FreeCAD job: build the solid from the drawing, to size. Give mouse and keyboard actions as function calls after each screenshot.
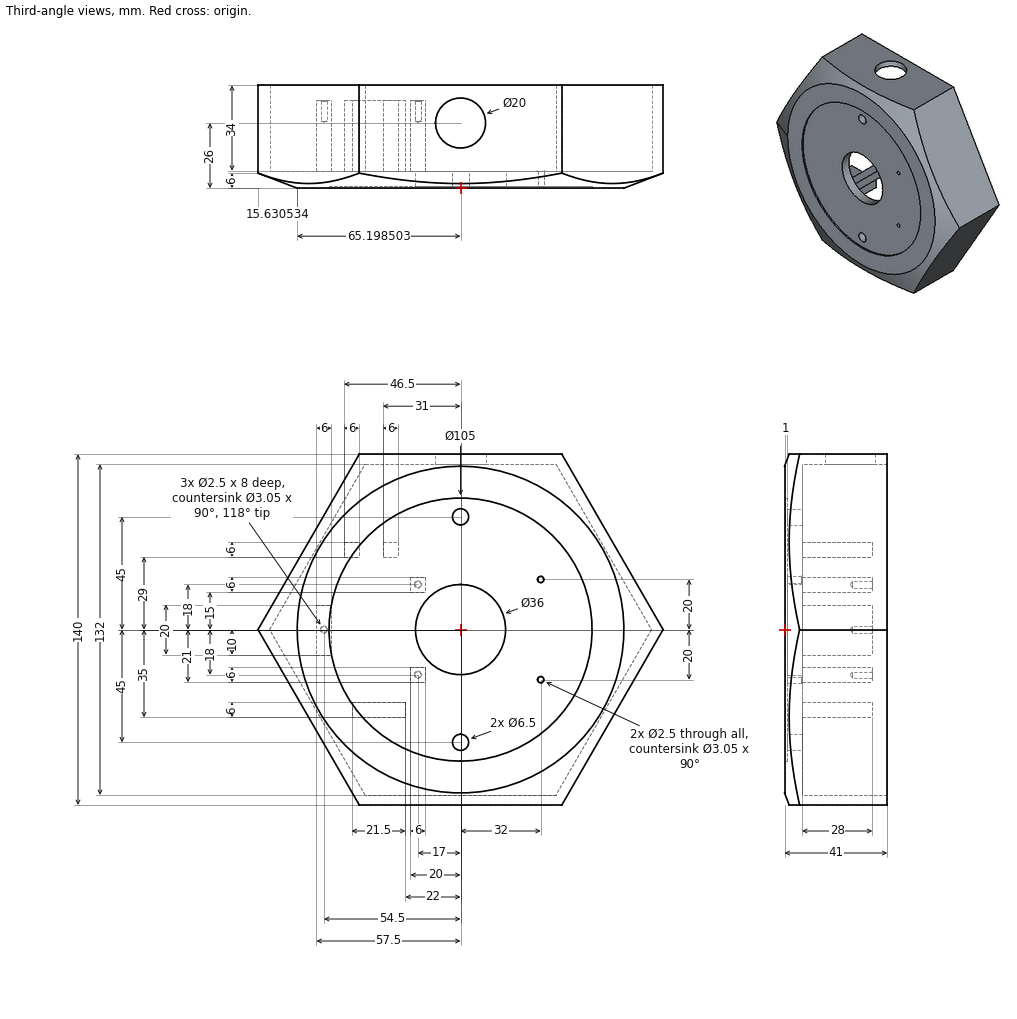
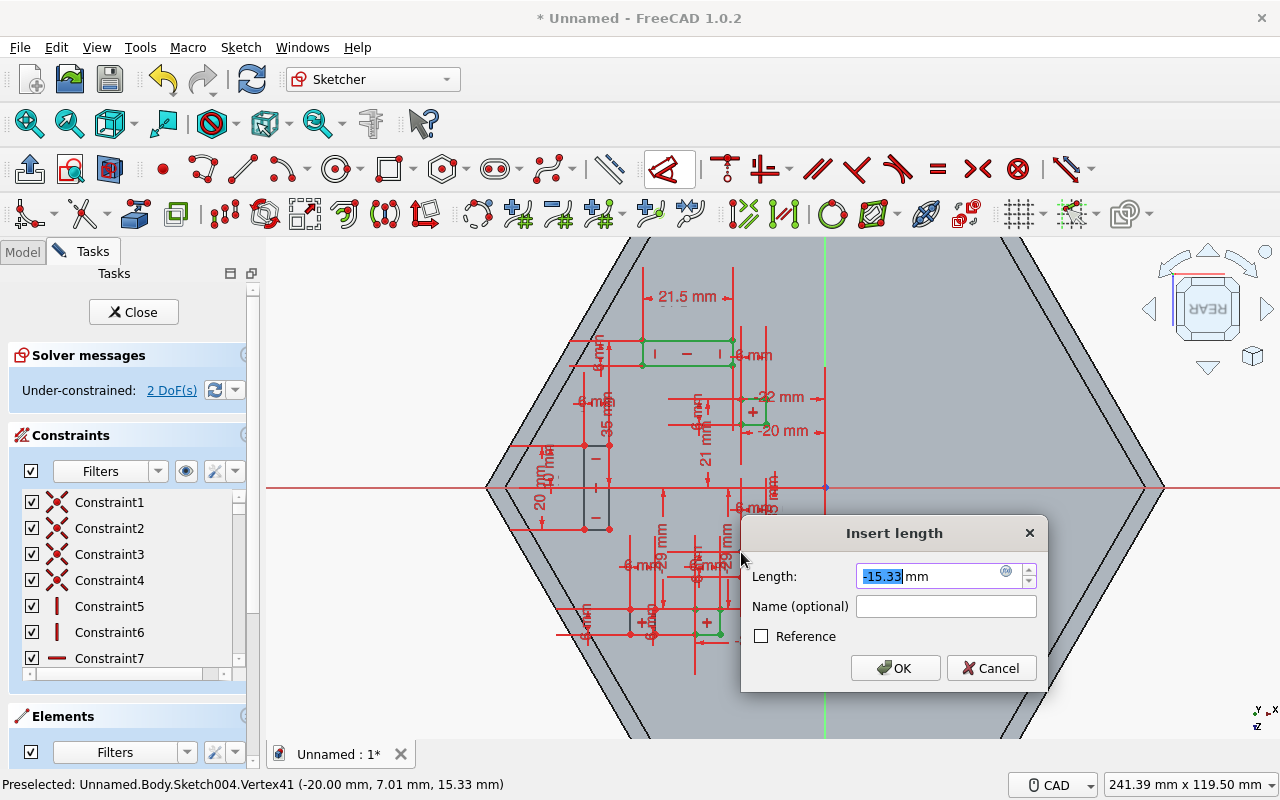
text(-15)
key(Return)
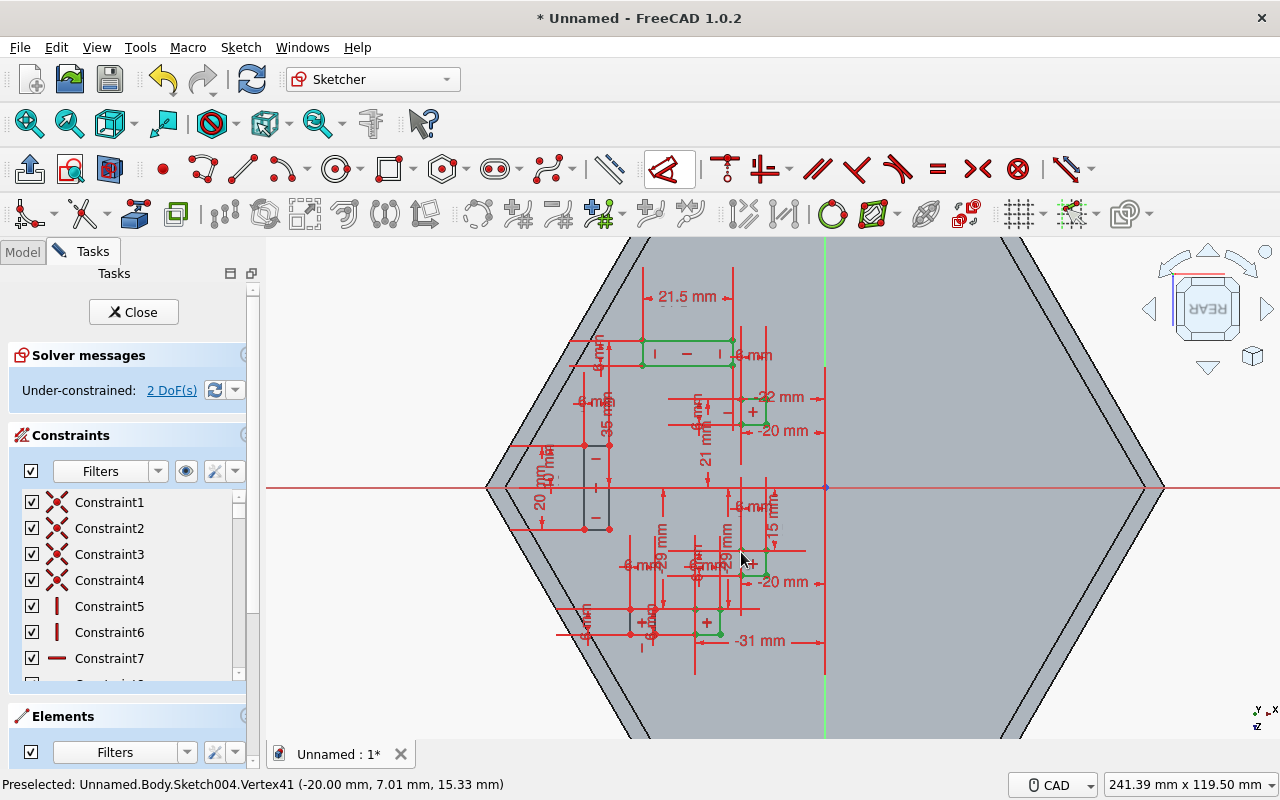
click(584, 446)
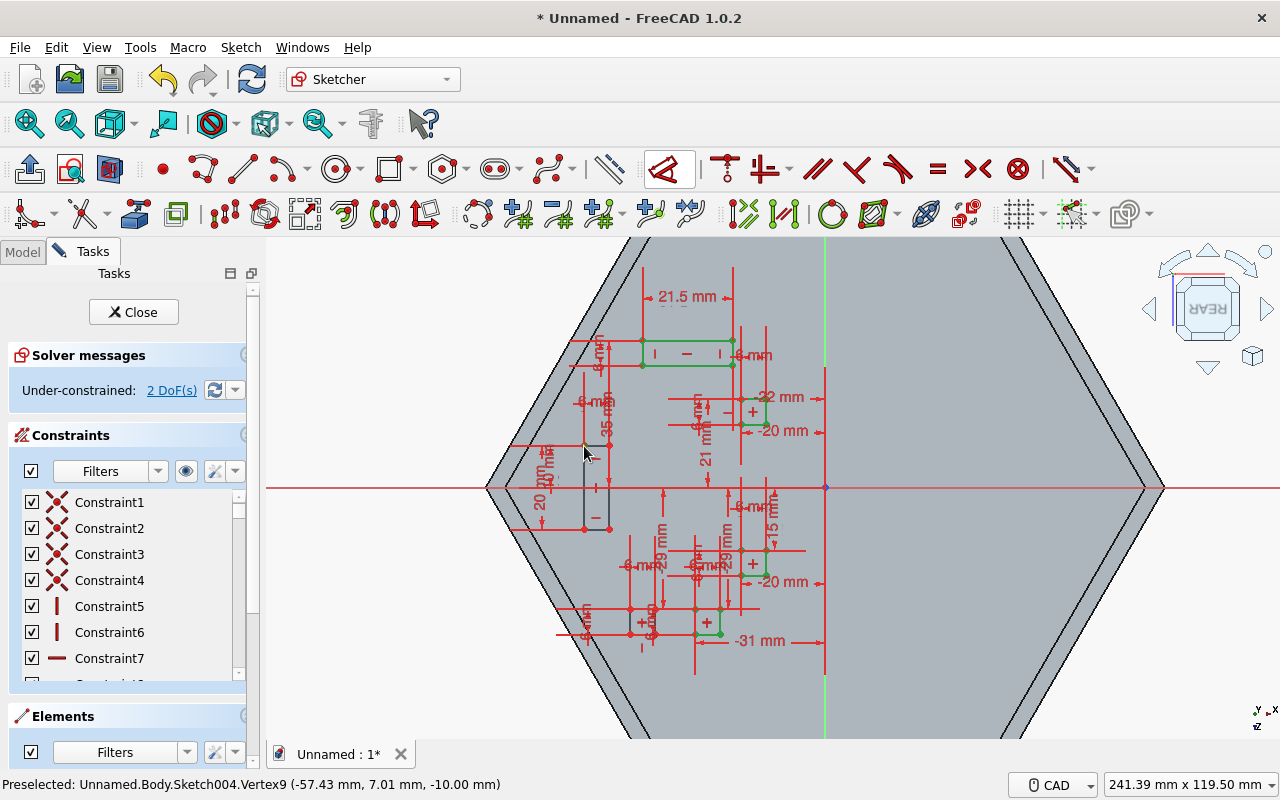
key(l)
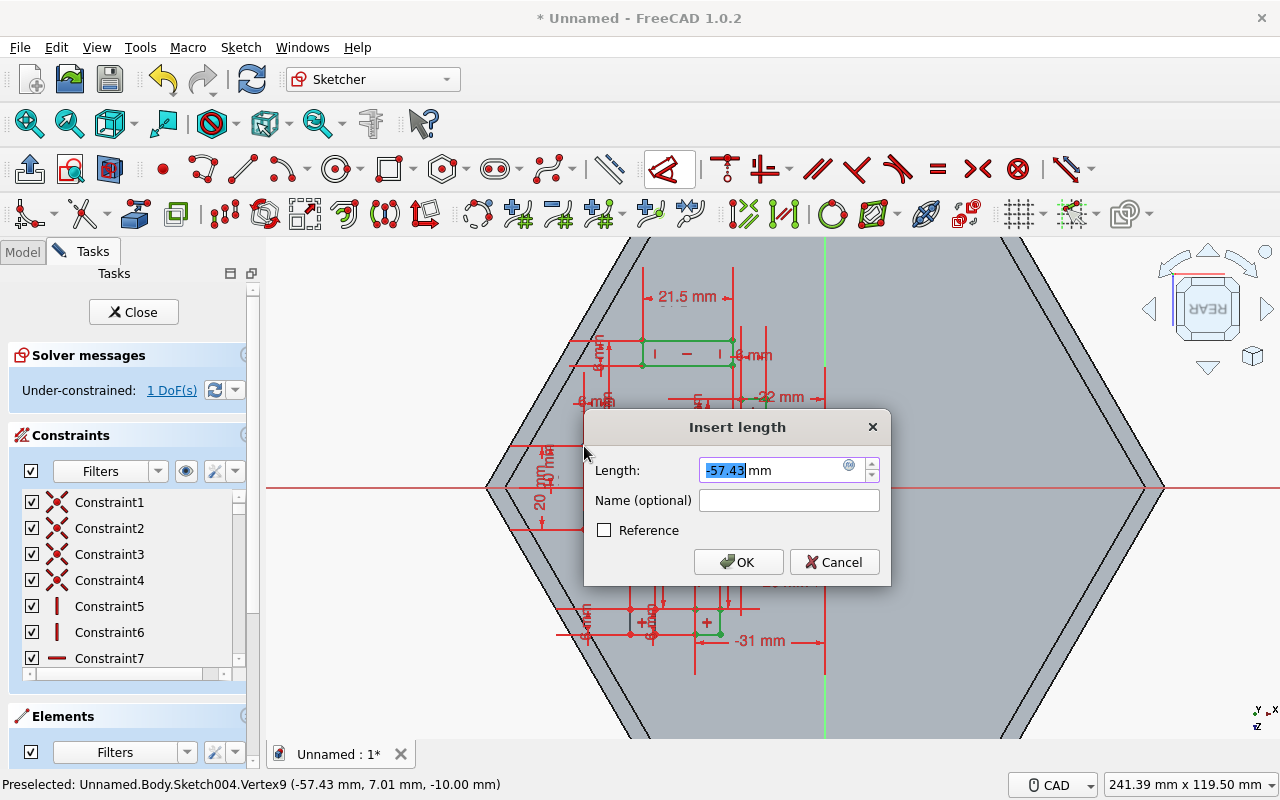
text(-57.5)
key(Return)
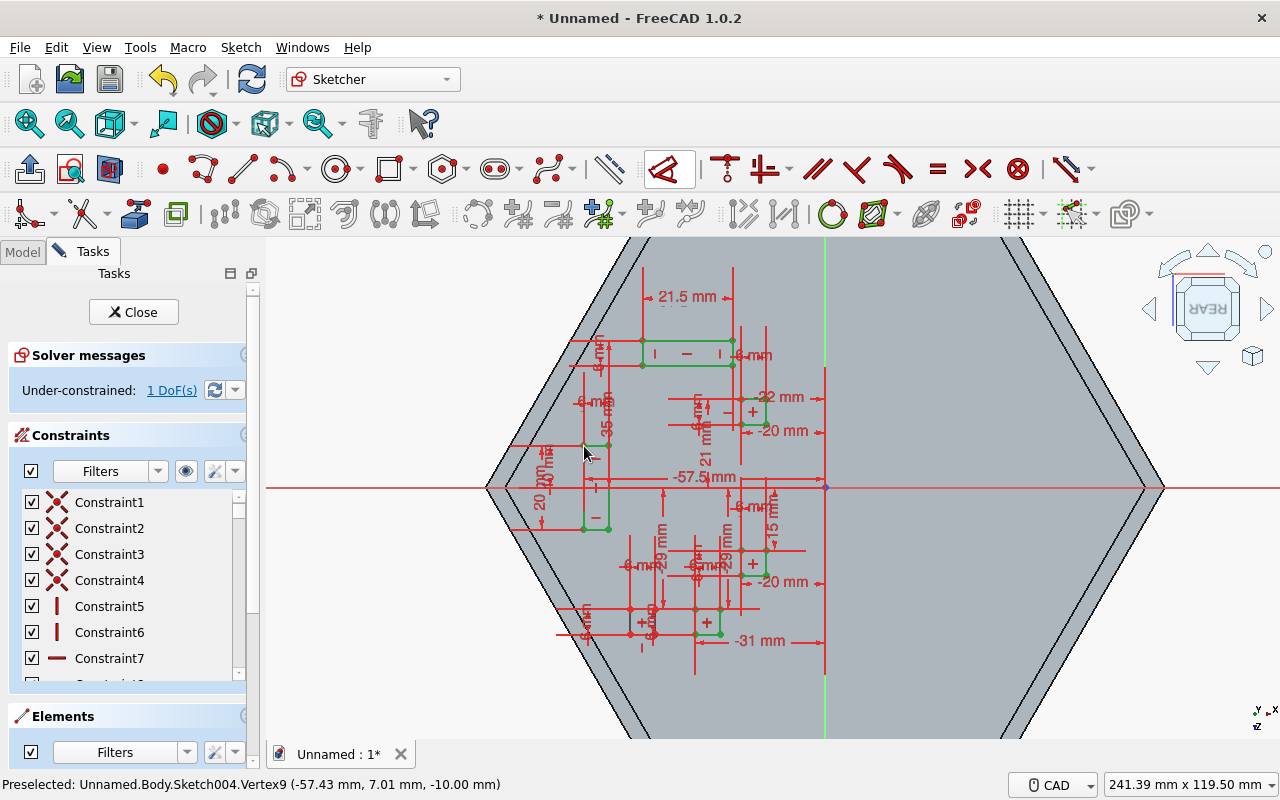
click(630, 609)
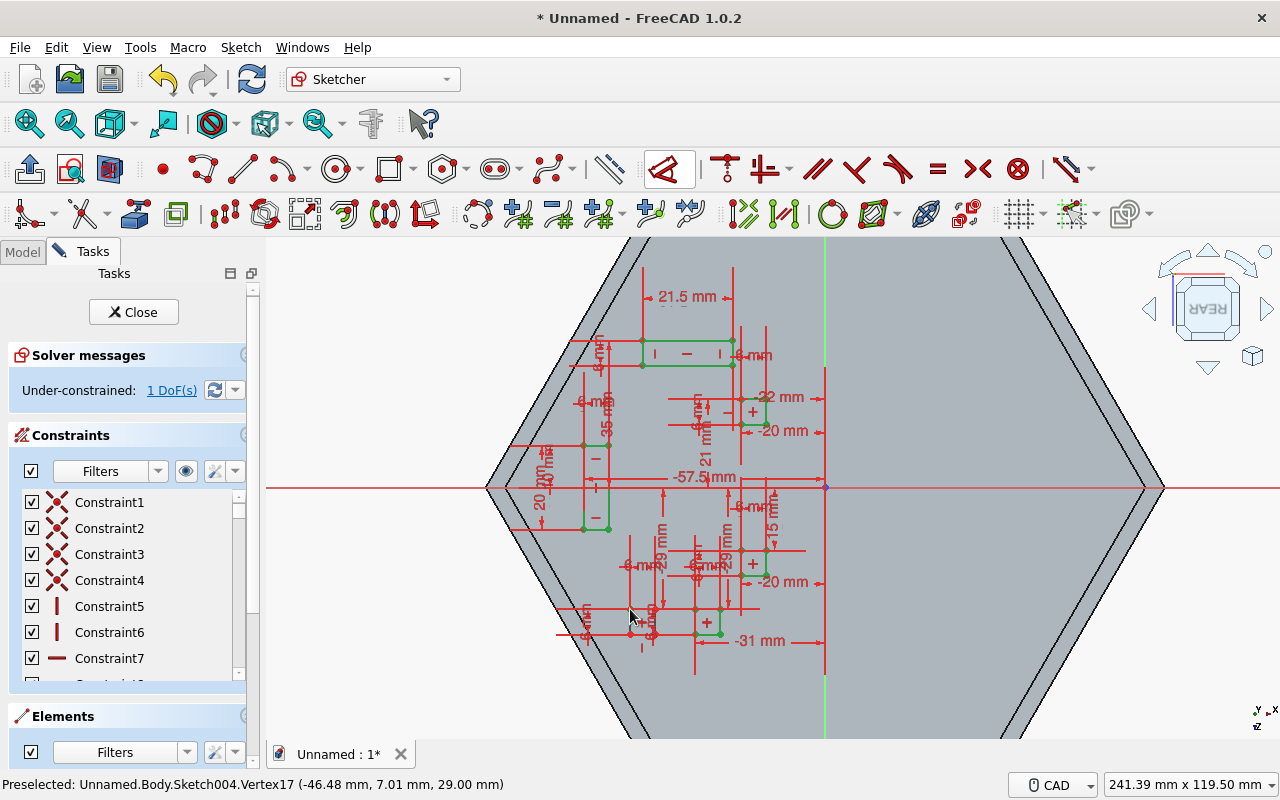
key(l)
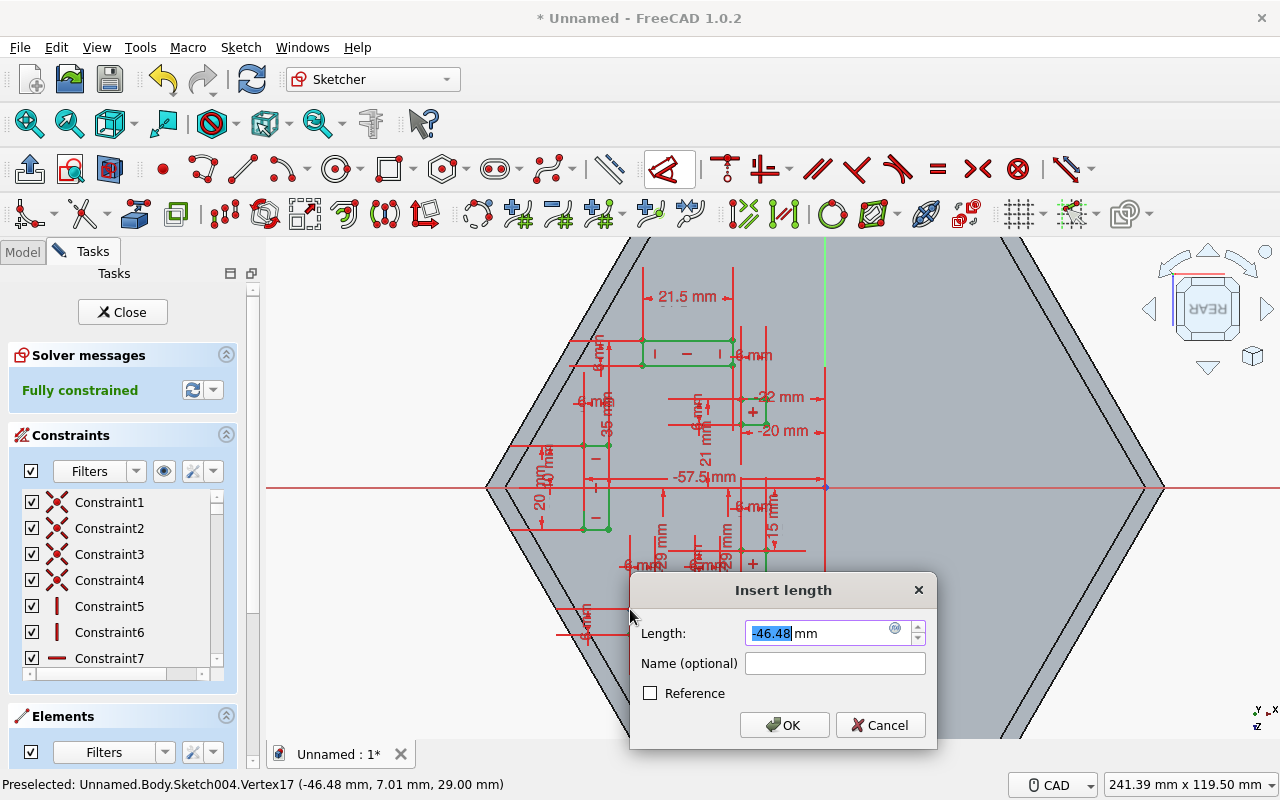
text(-46.5)
key(Return)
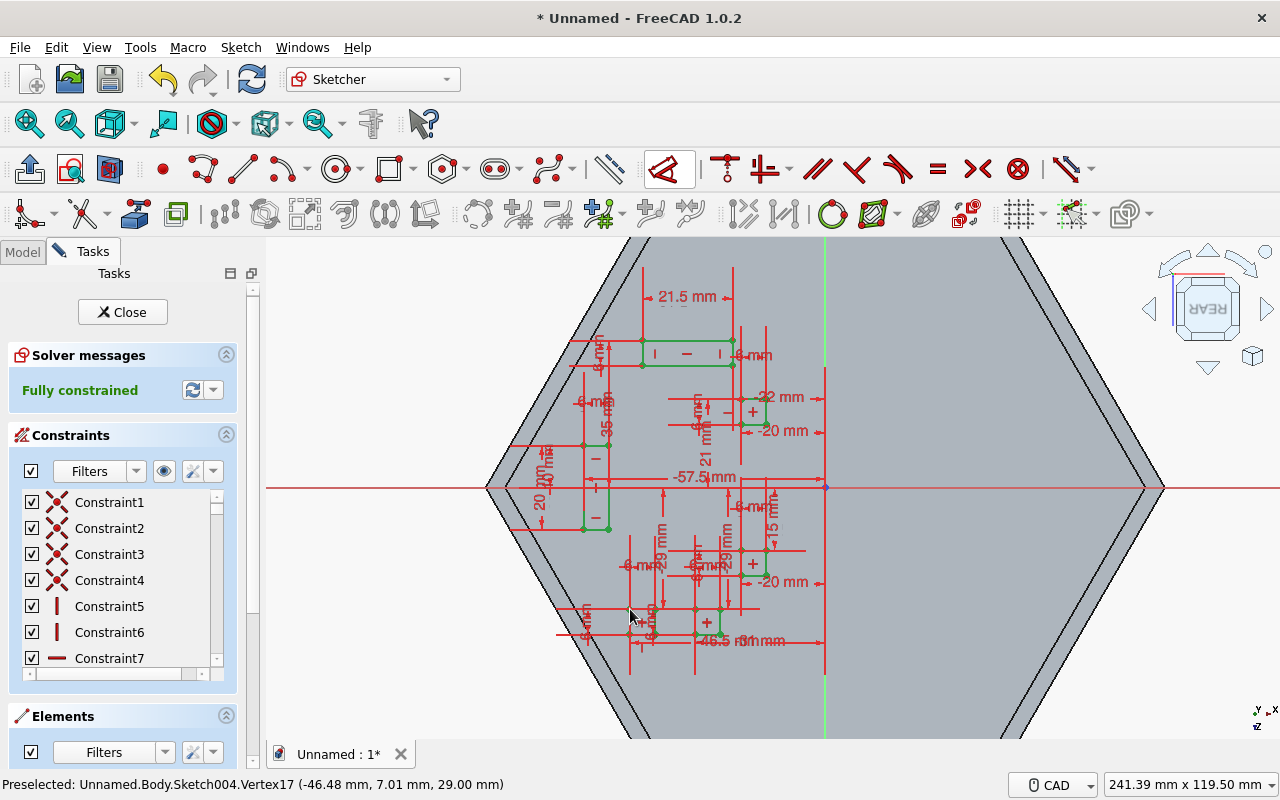
click(123, 312)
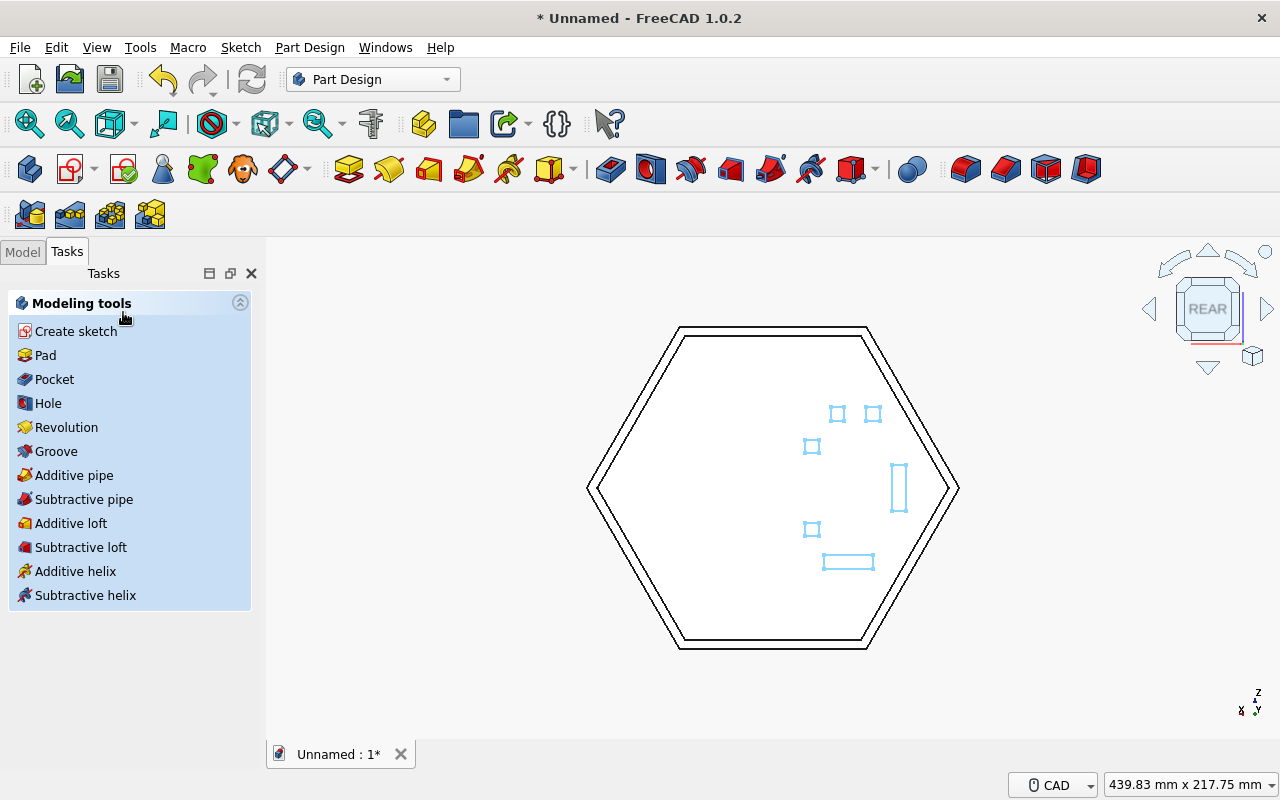
click(350, 170)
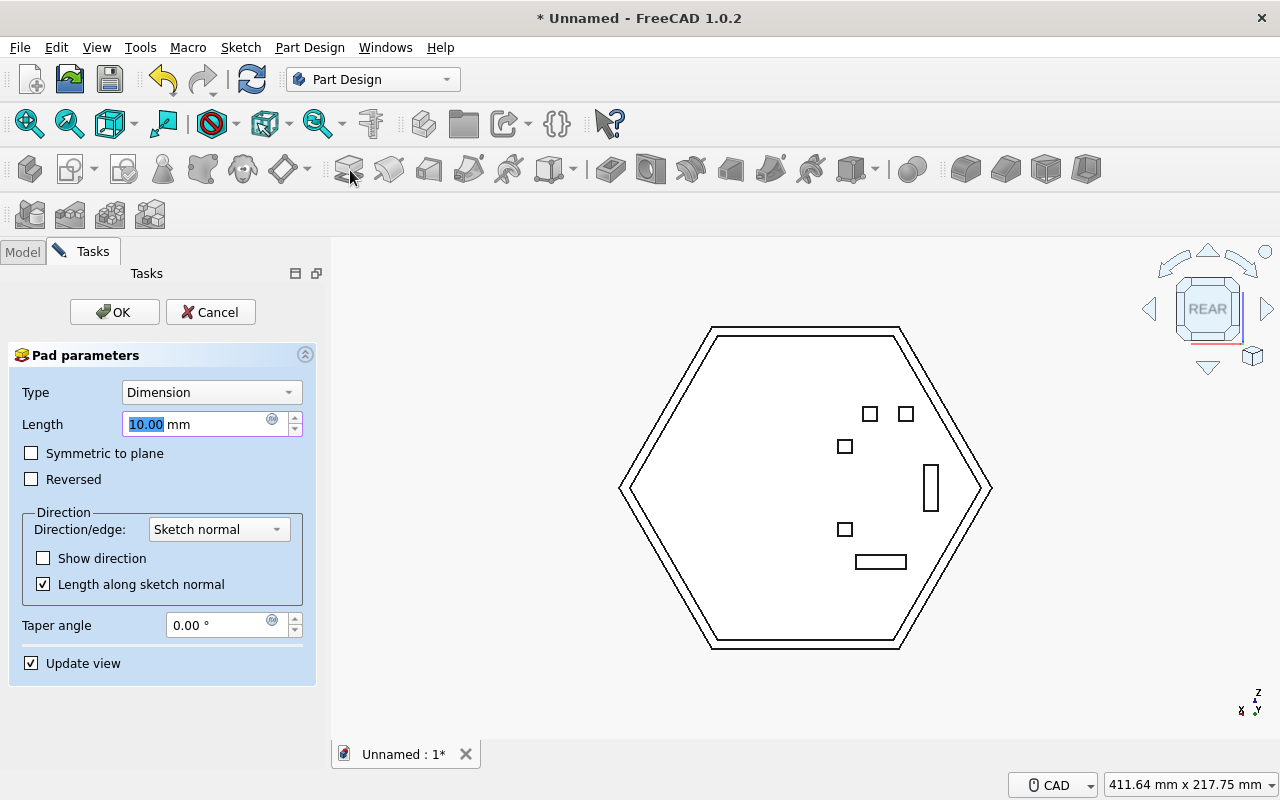
text(28)
key(Tab)